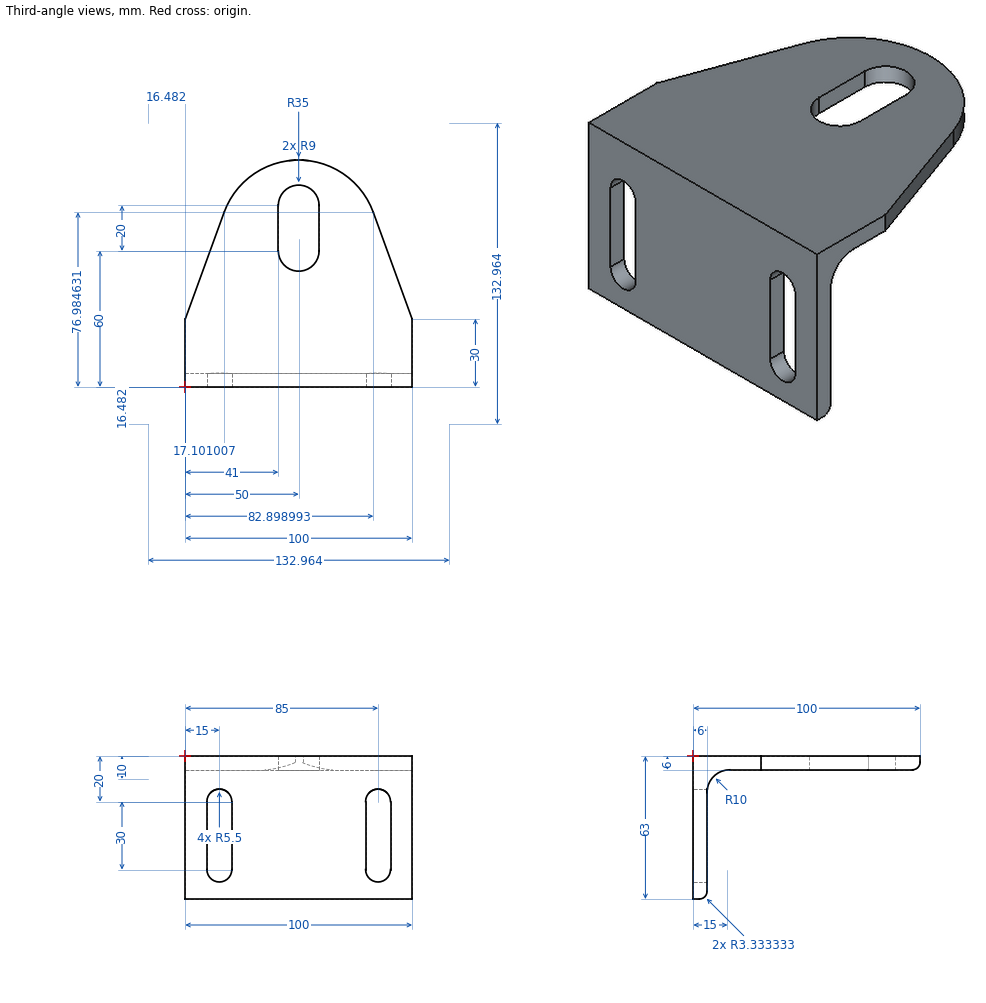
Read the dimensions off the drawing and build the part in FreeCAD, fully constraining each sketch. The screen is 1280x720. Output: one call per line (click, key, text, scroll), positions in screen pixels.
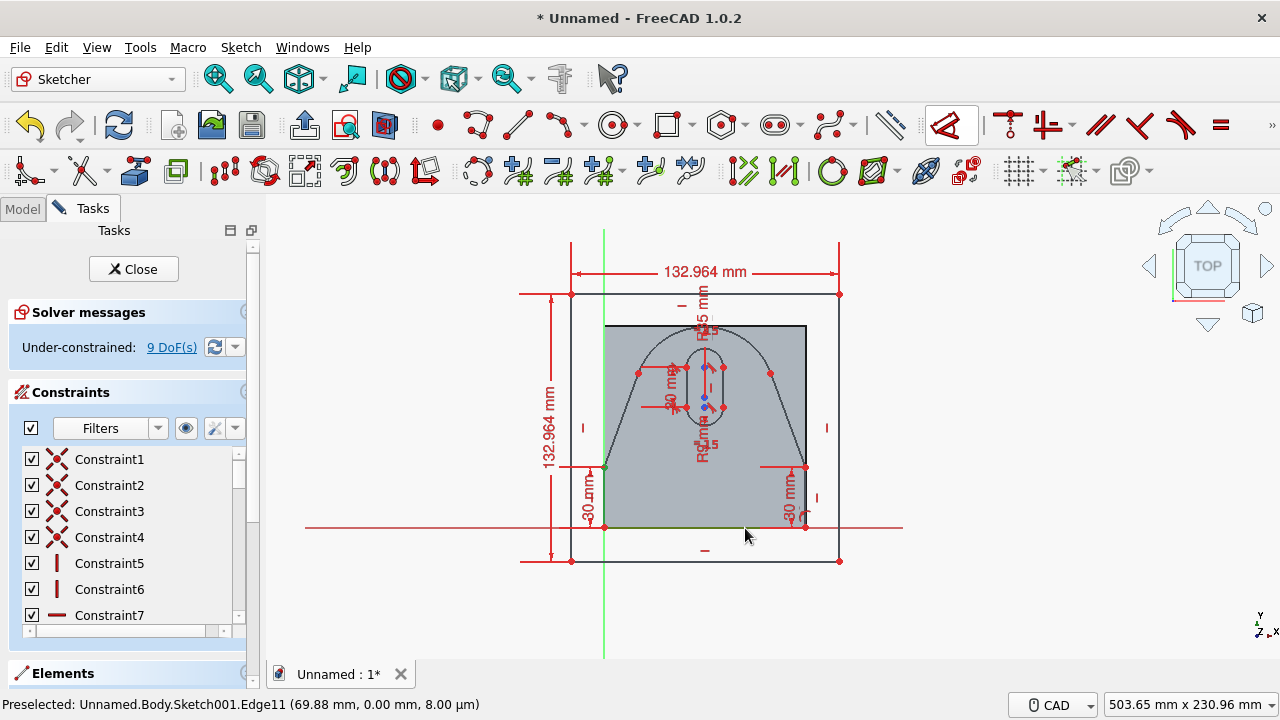
click(972, 126)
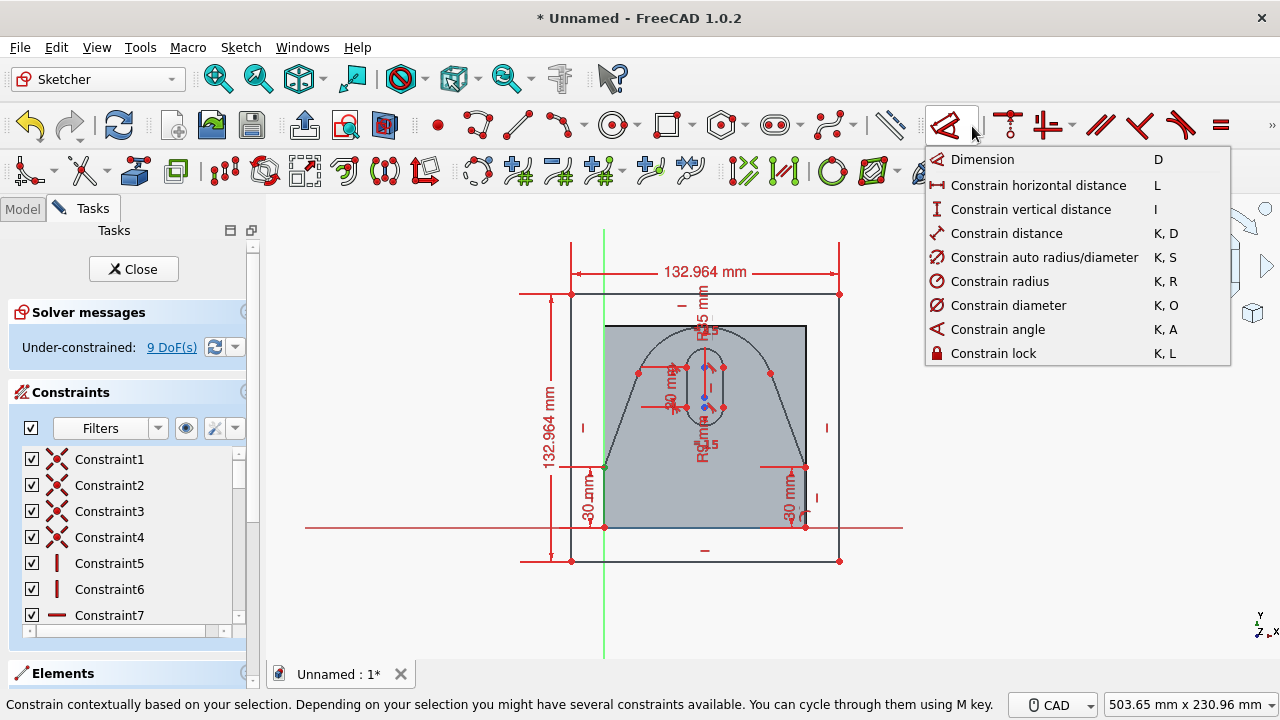
click(1078, 185)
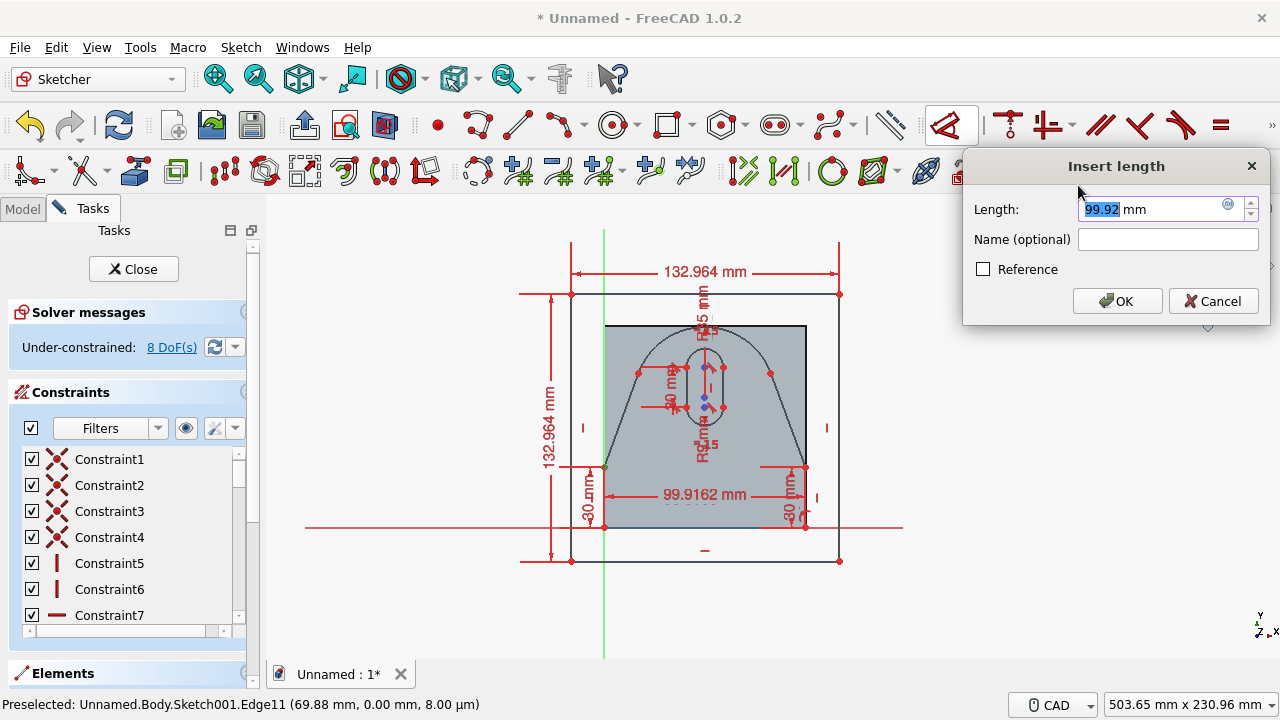
text(100)
key(Return)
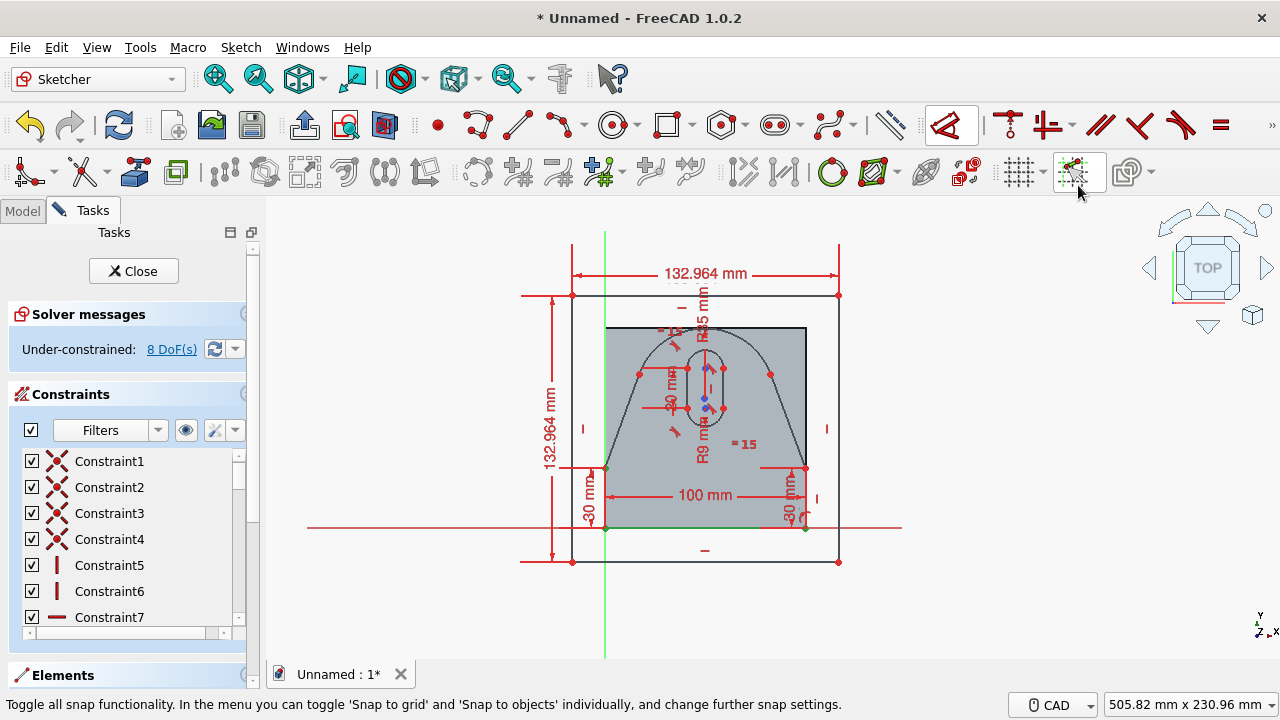
click(687, 408)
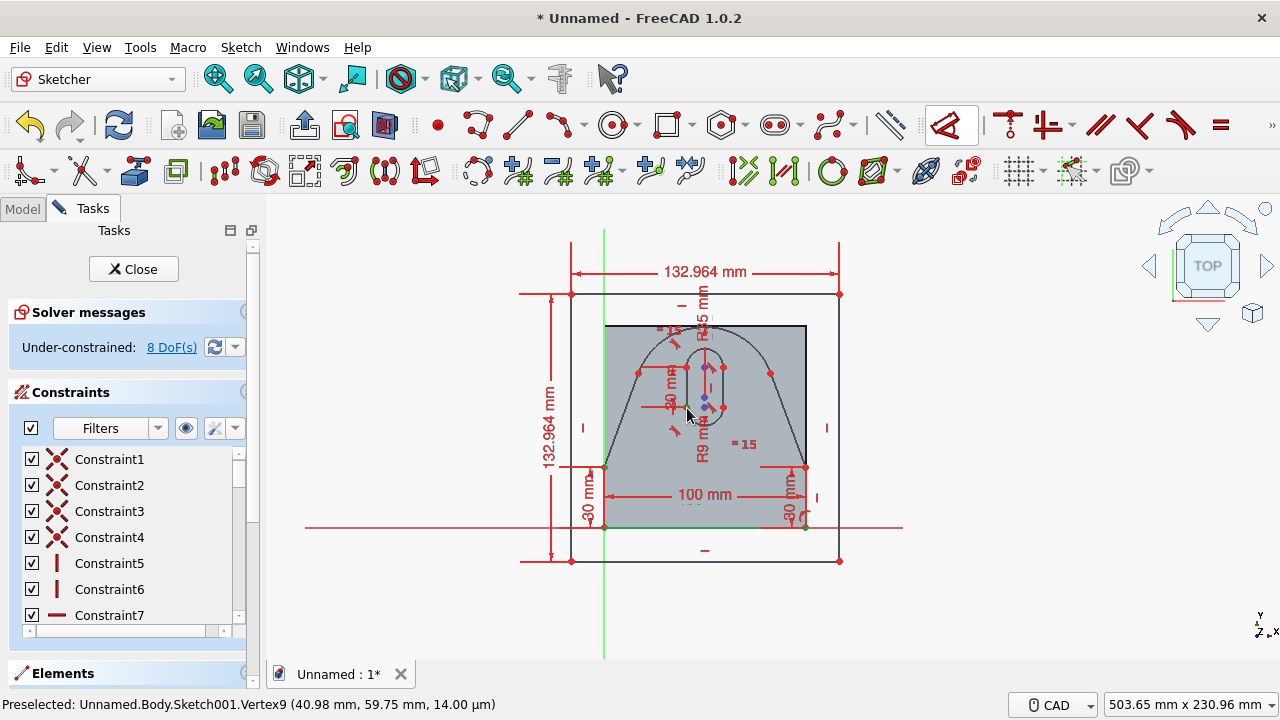
click(972, 126)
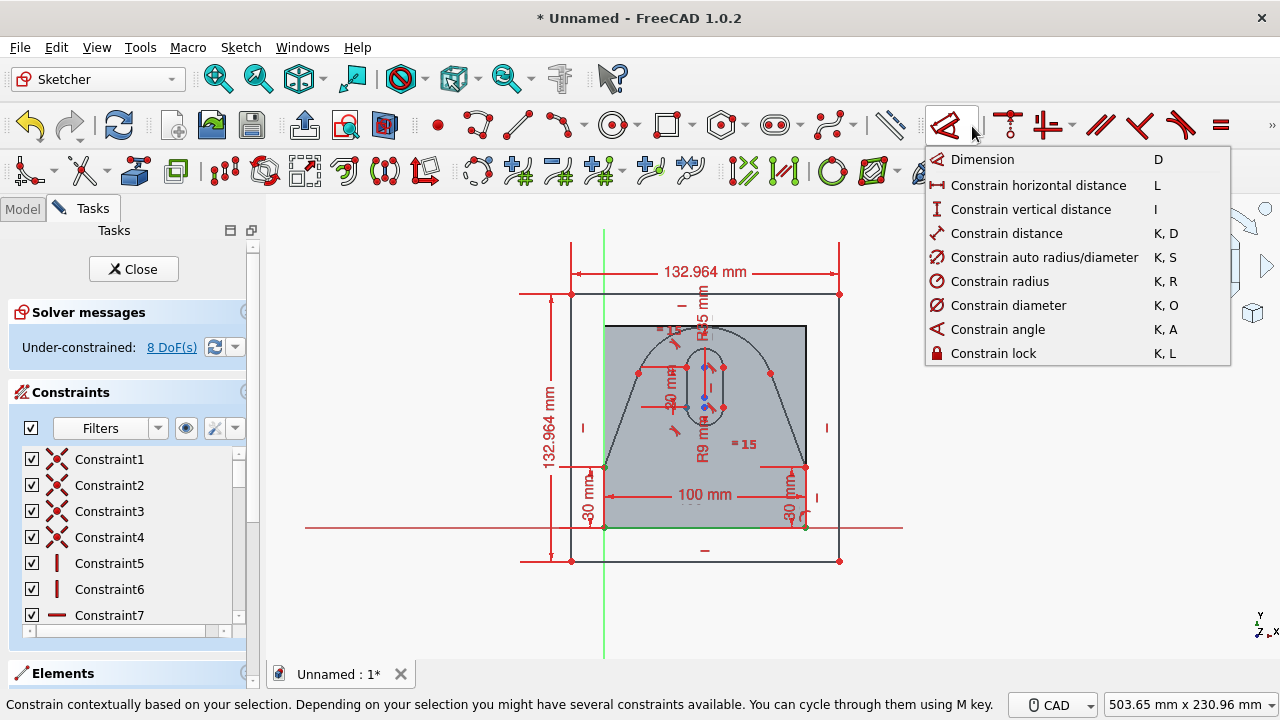
click(1078, 185)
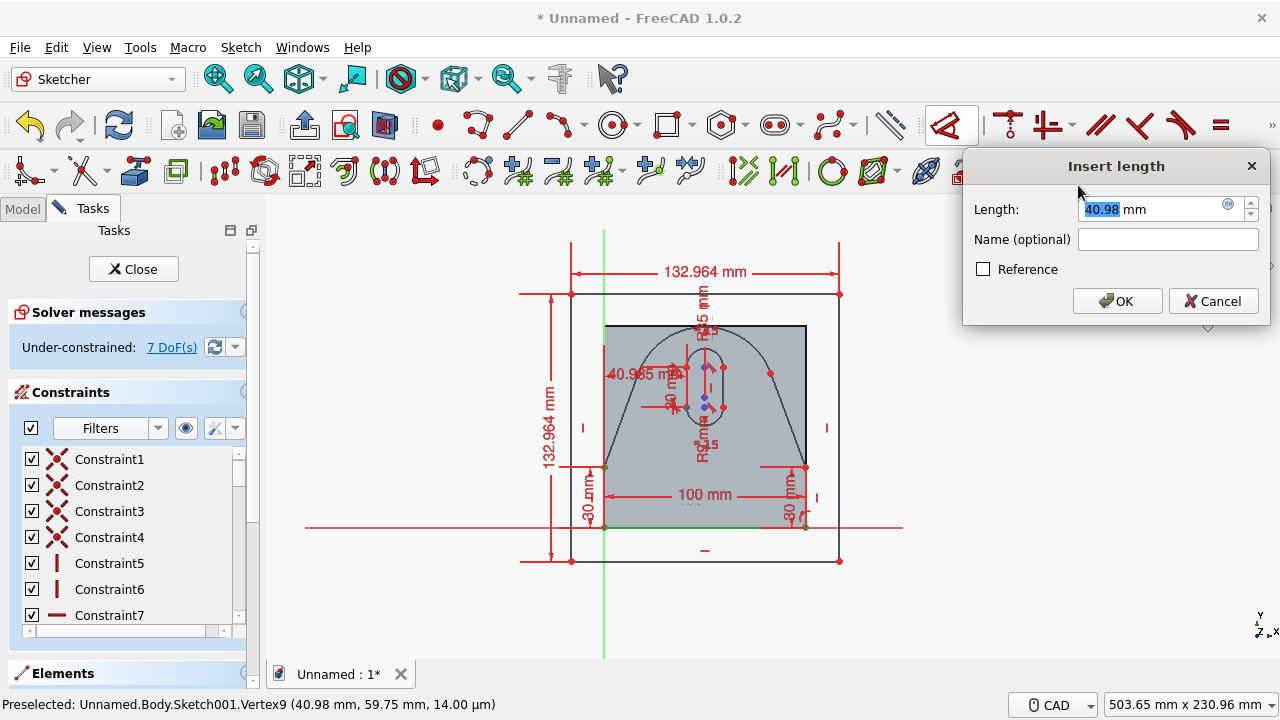
text(41)
key(Return)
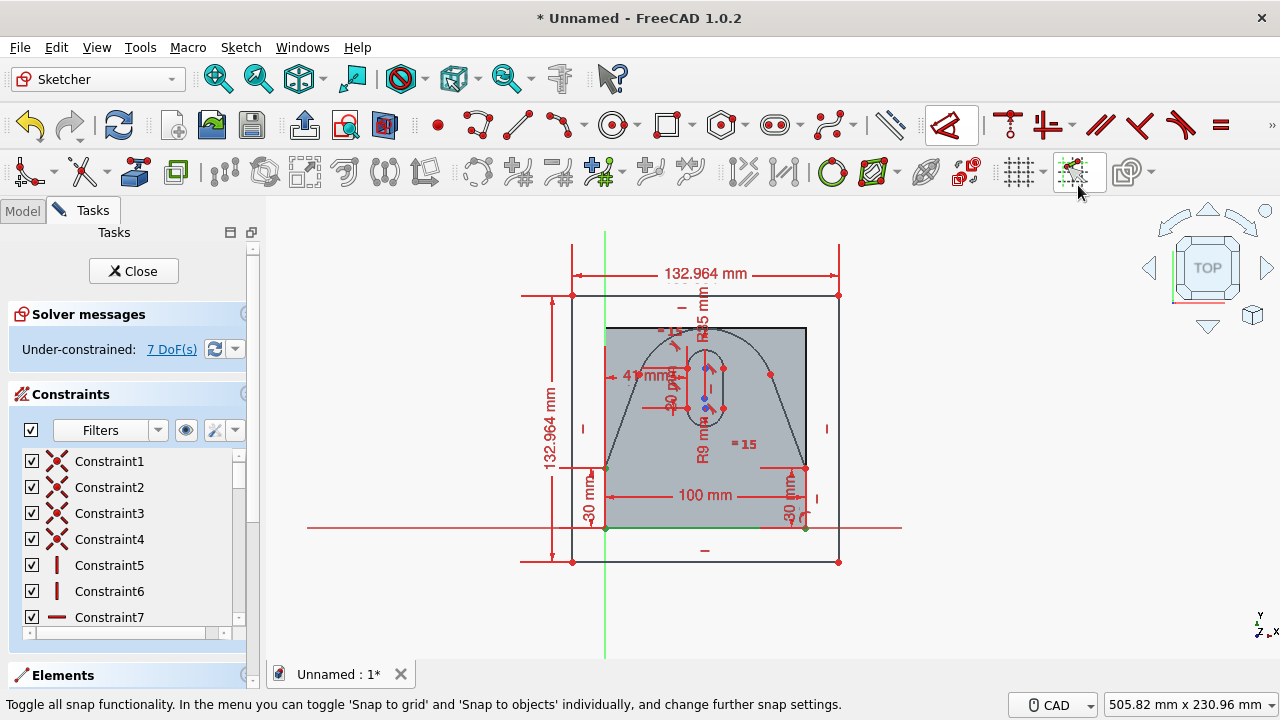
click(687, 408)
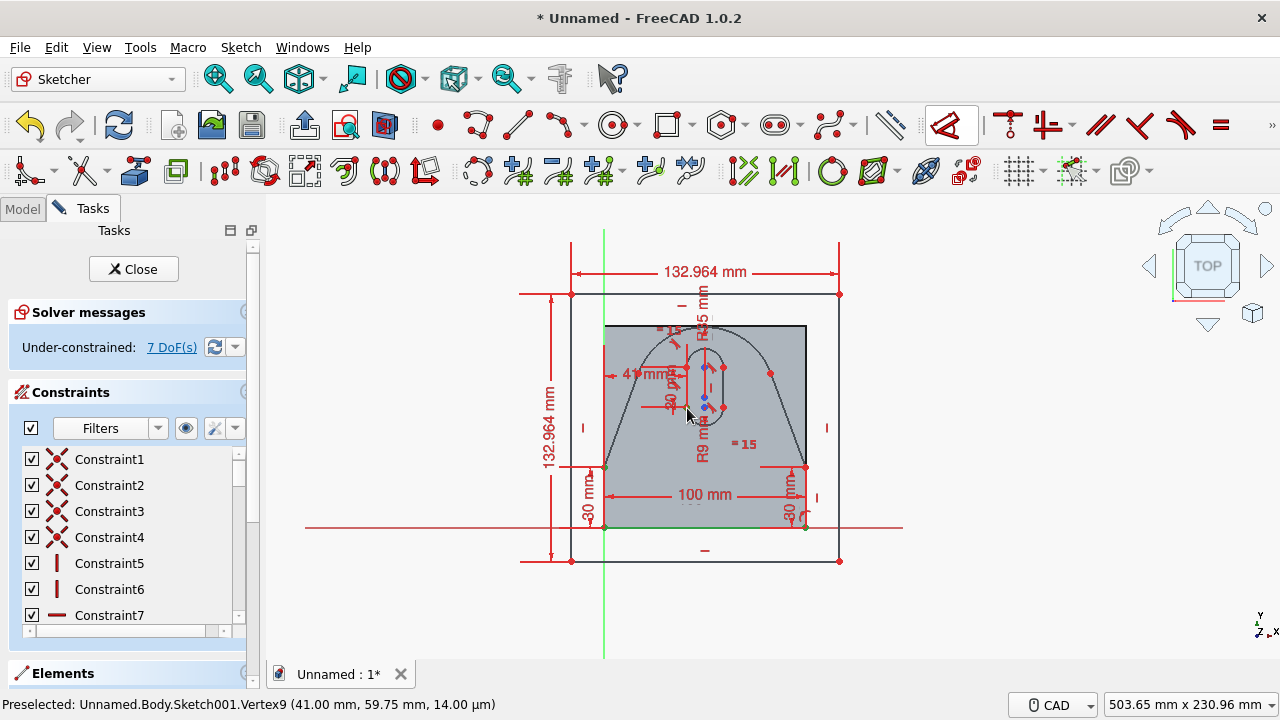
key(i)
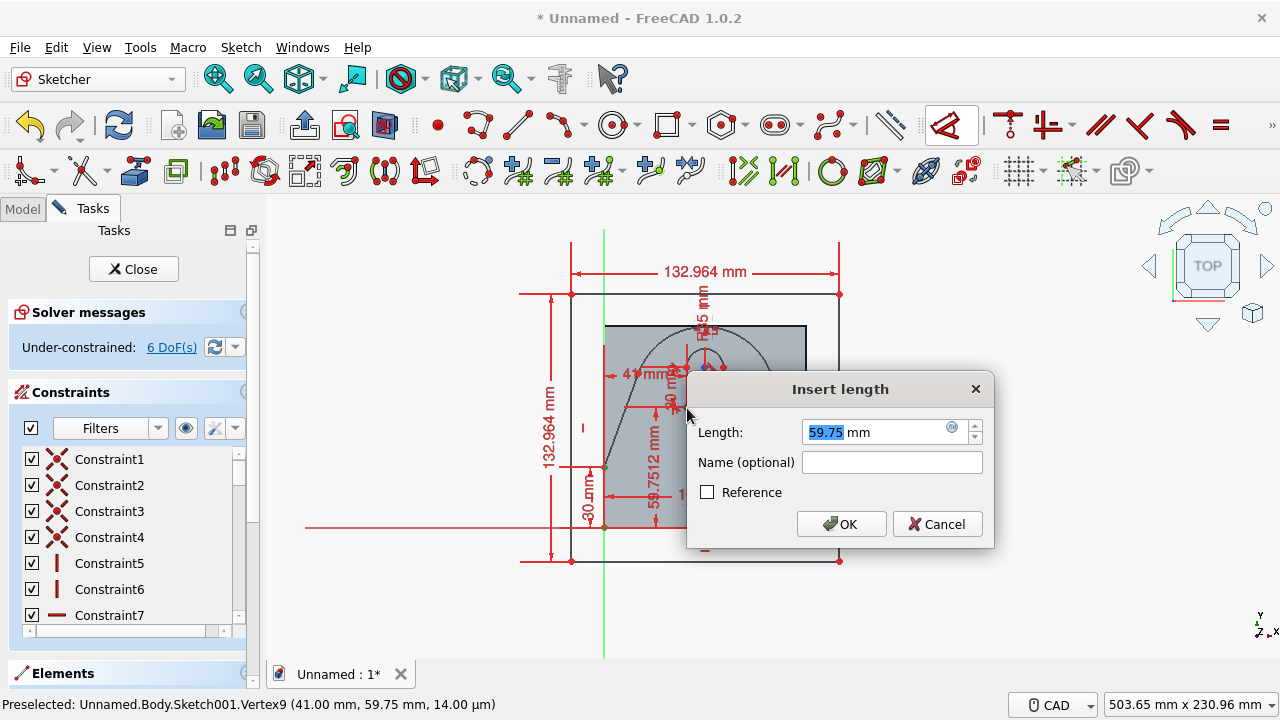
text(60)
key(Return)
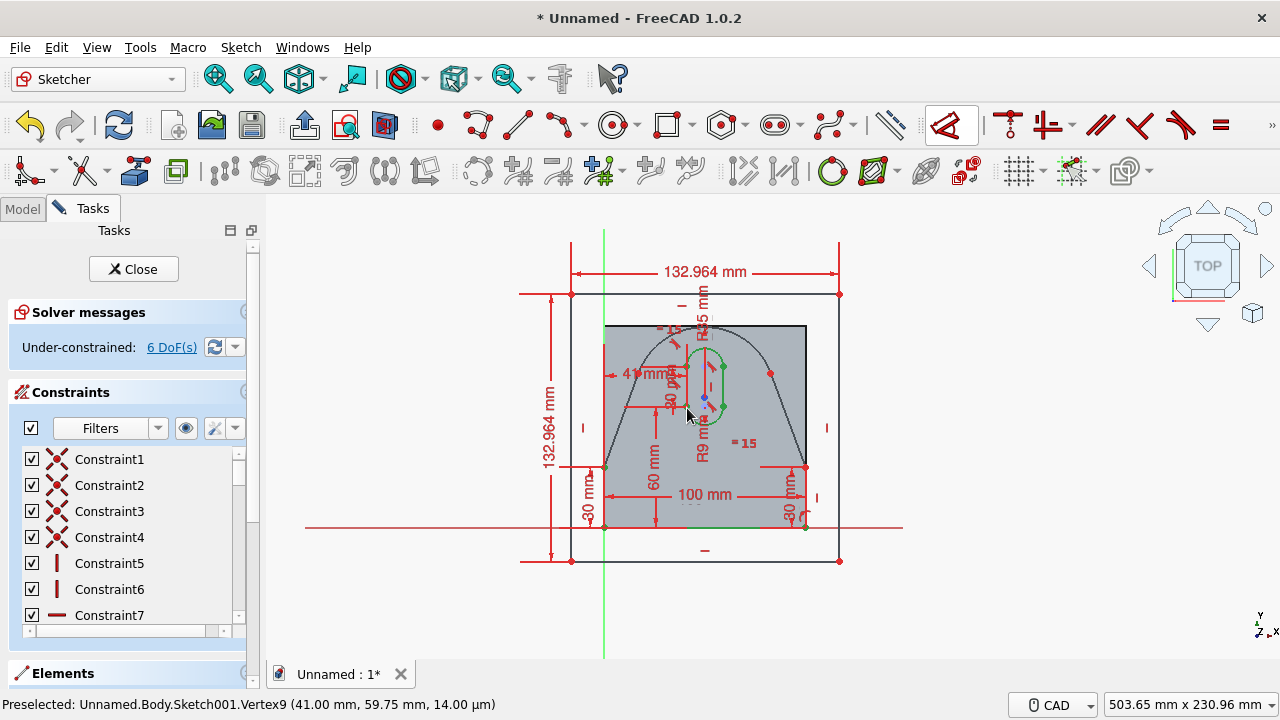
scroll(705, 398, up, 2)